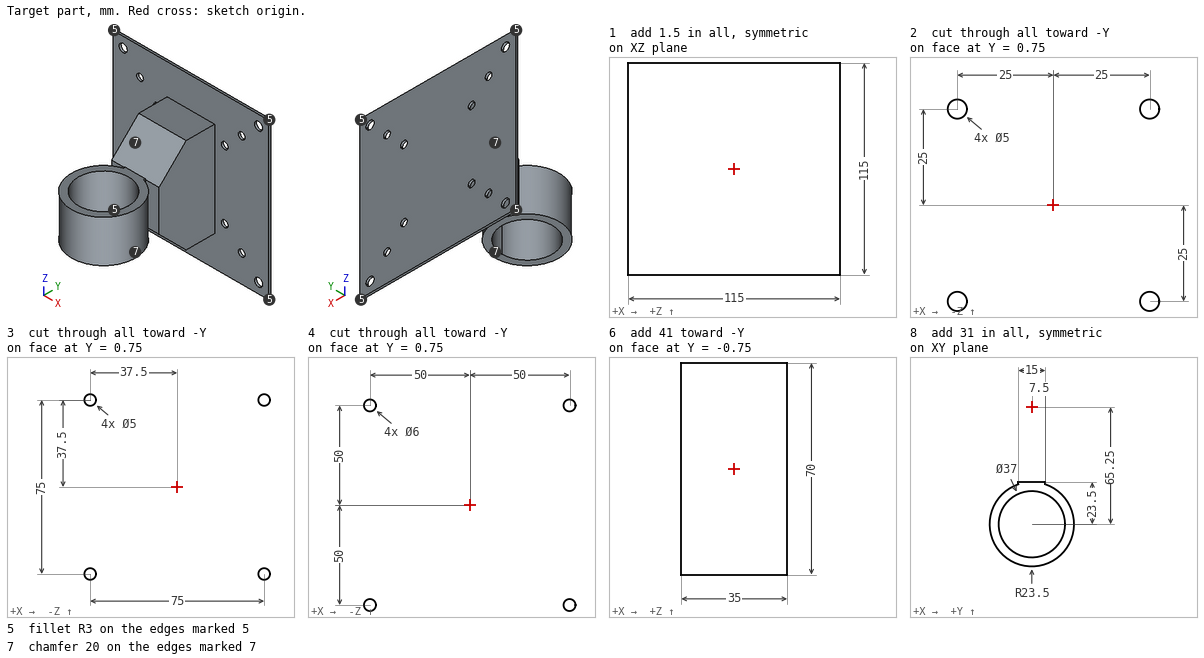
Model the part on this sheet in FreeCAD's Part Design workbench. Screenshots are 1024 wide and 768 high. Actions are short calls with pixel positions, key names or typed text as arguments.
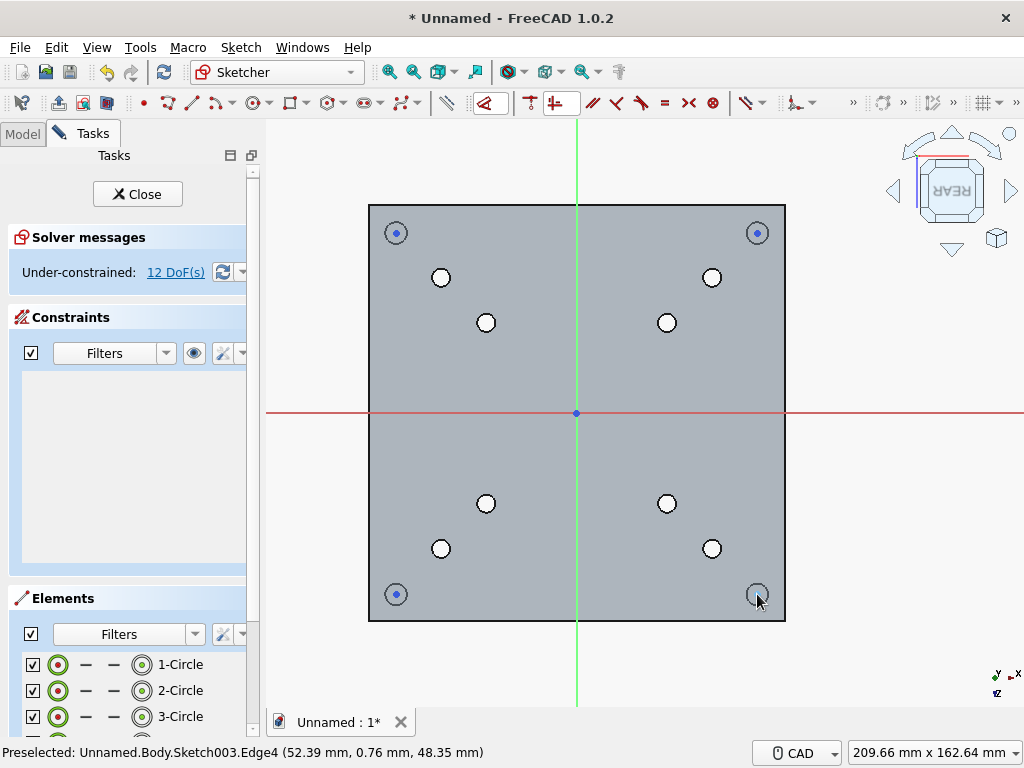
scroll(404, 225, up, 2)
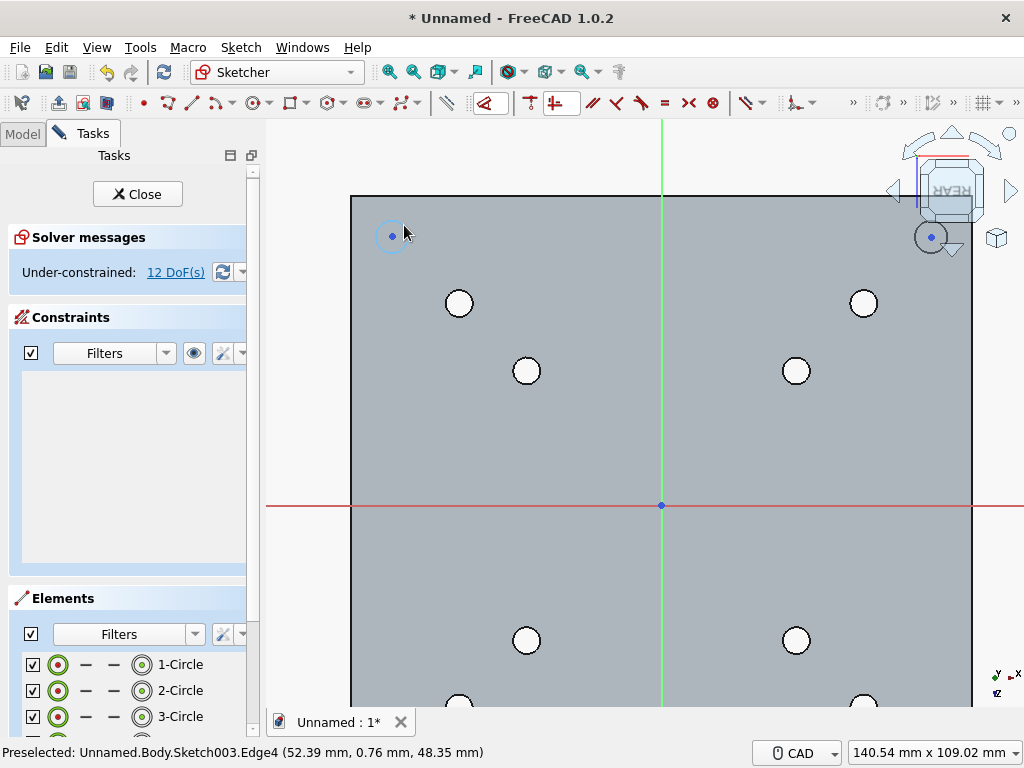
click(403, 225)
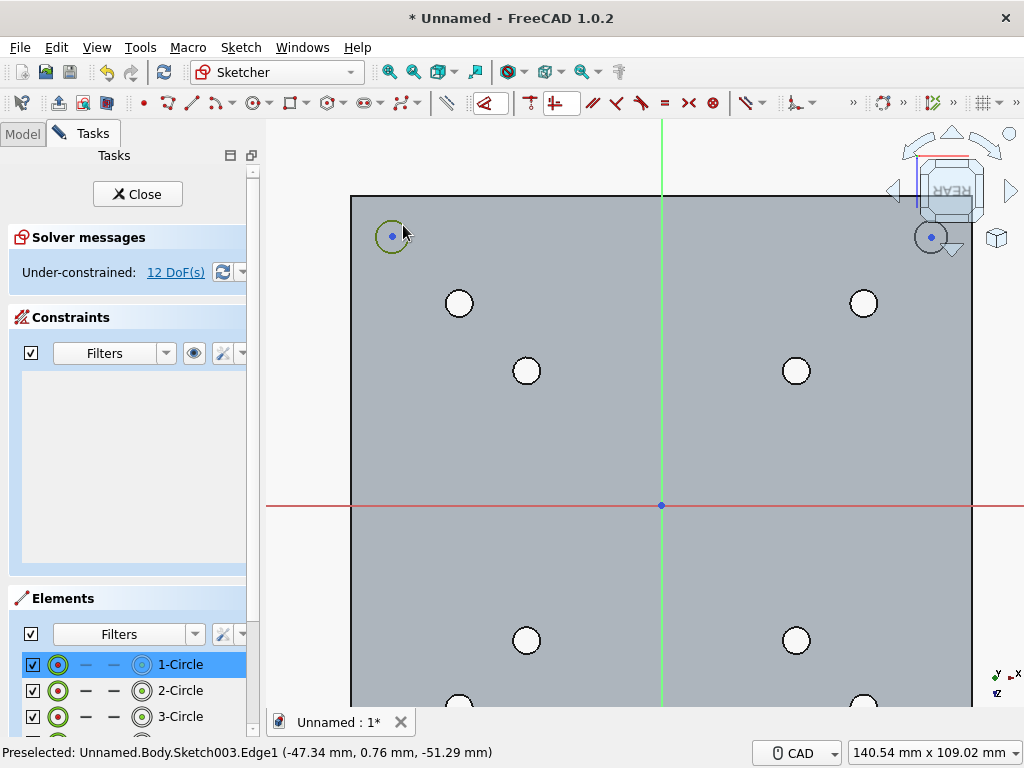
scroll(404, 224, down, 2)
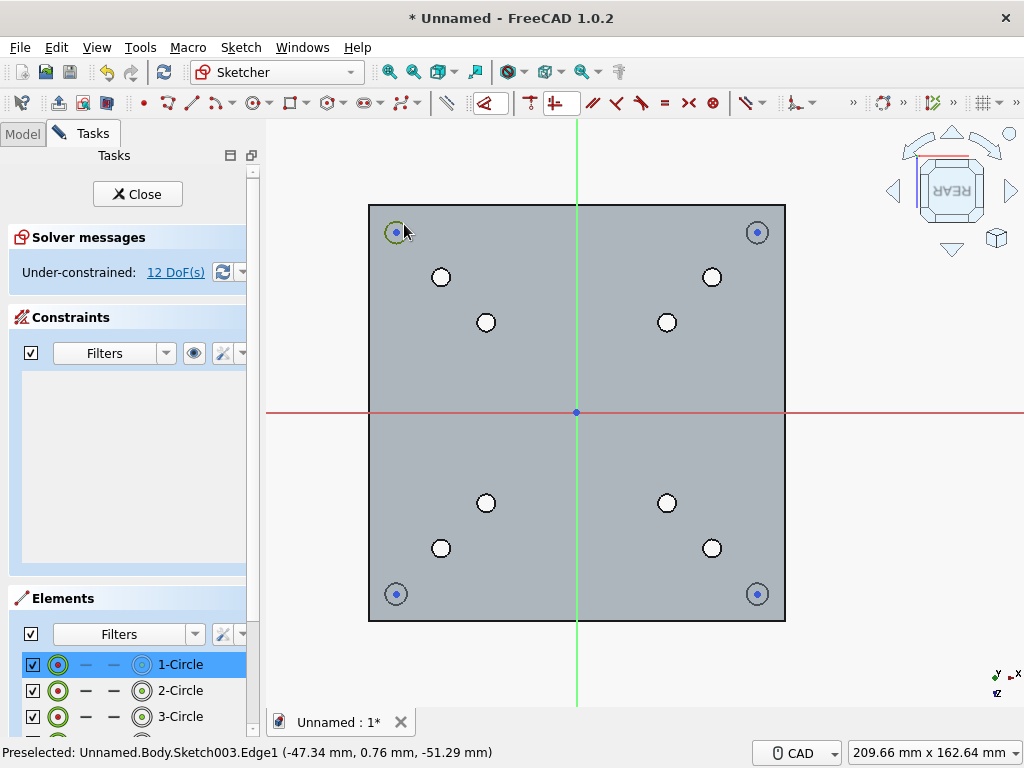
scroll(765, 225, up, 2)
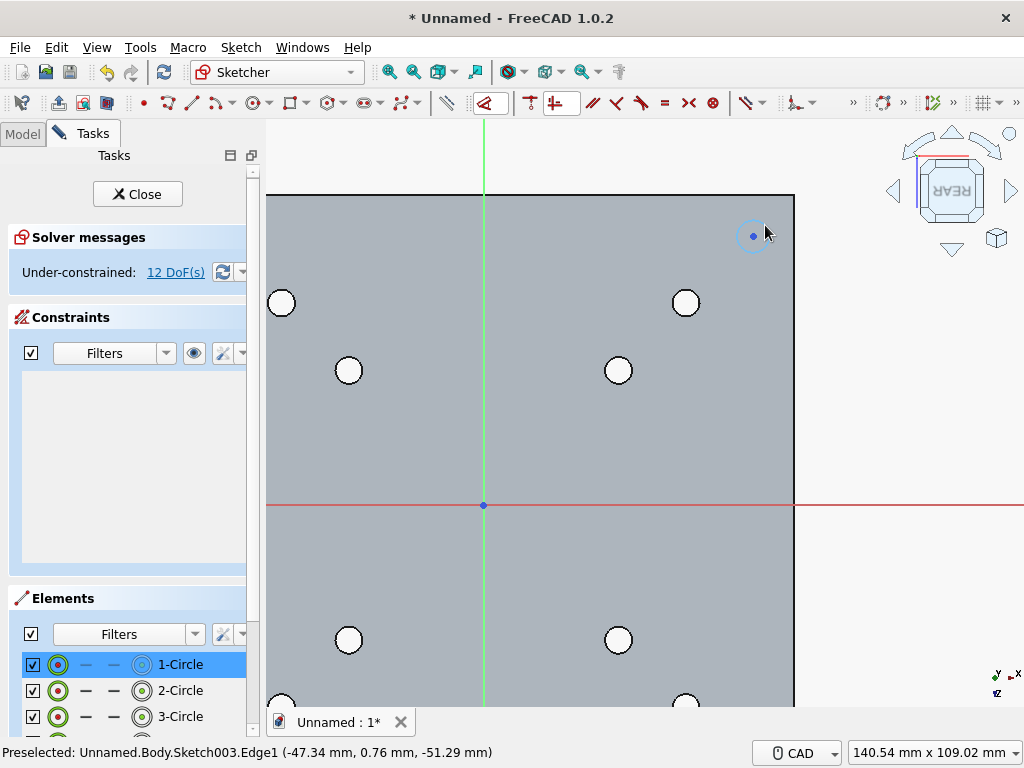
click(765, 225)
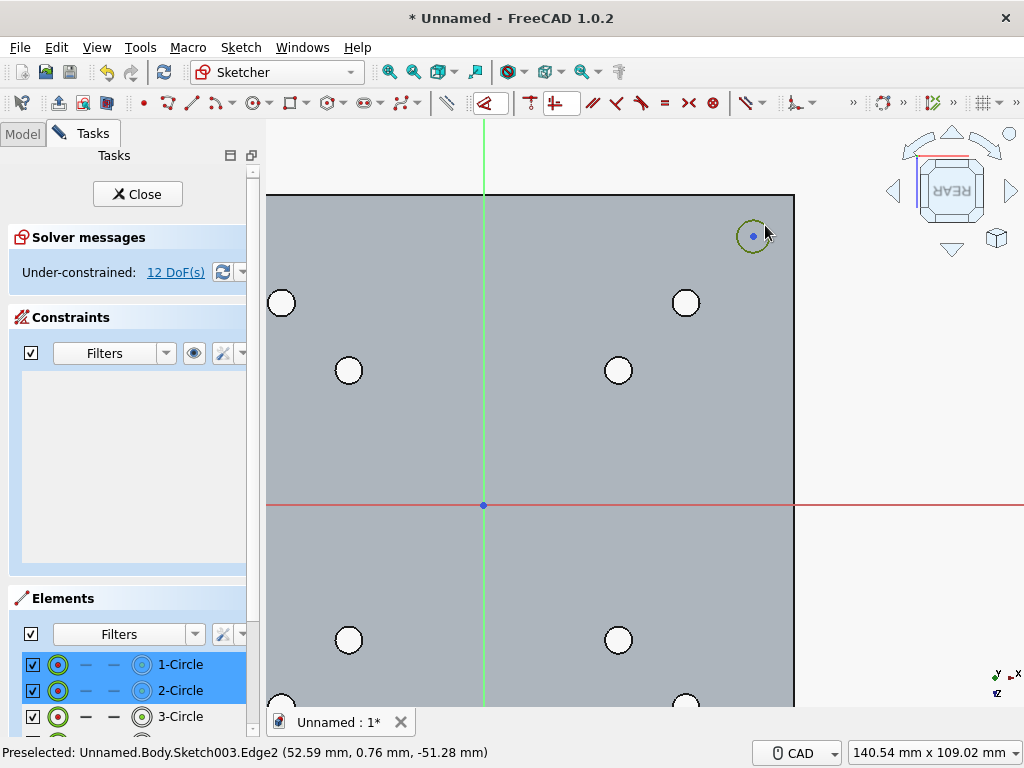
scroll(765, 225, down, 2)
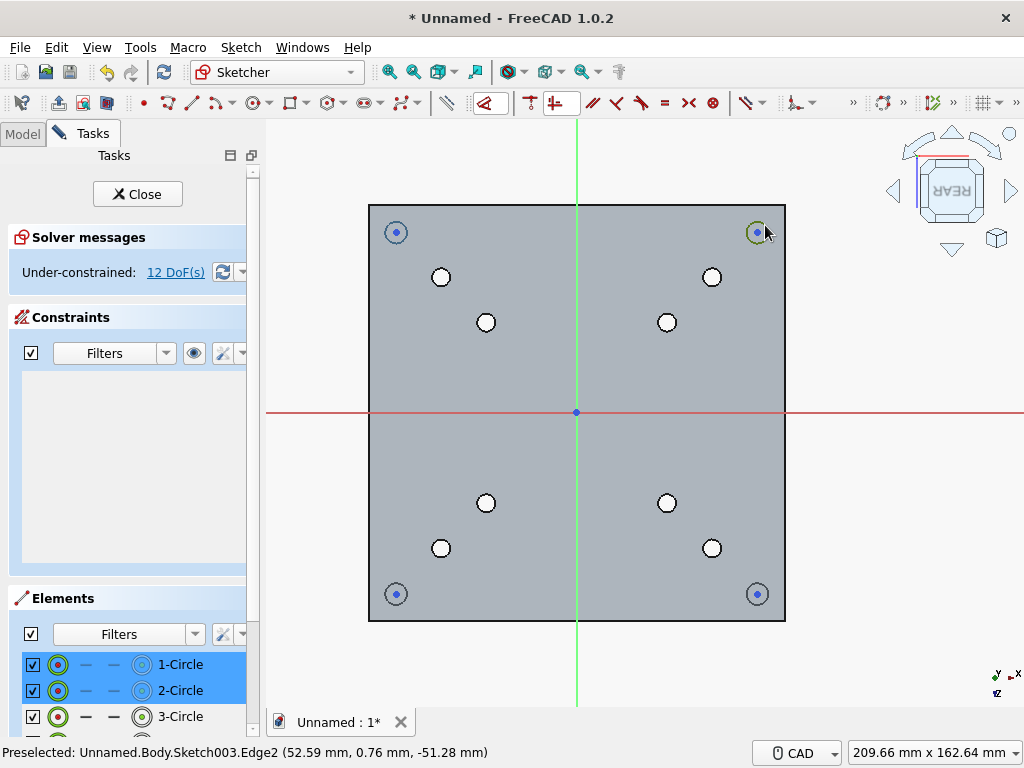
scroll(404, 586, up, 2)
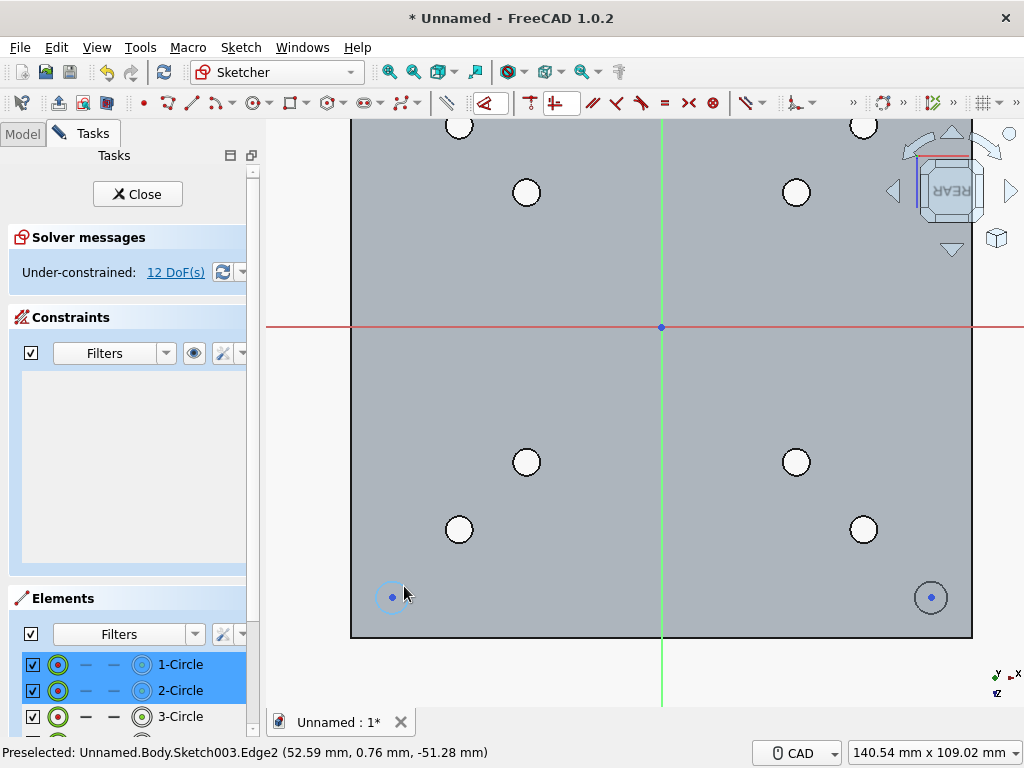
click(403, 586)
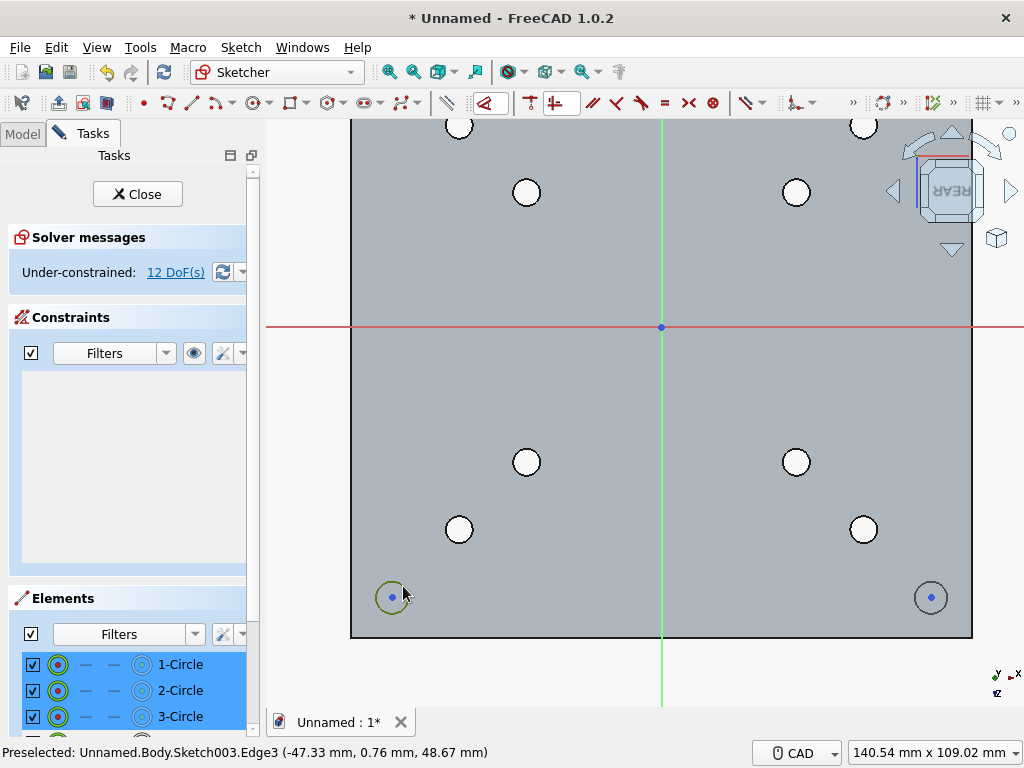
scroll(404, 587, down, 2)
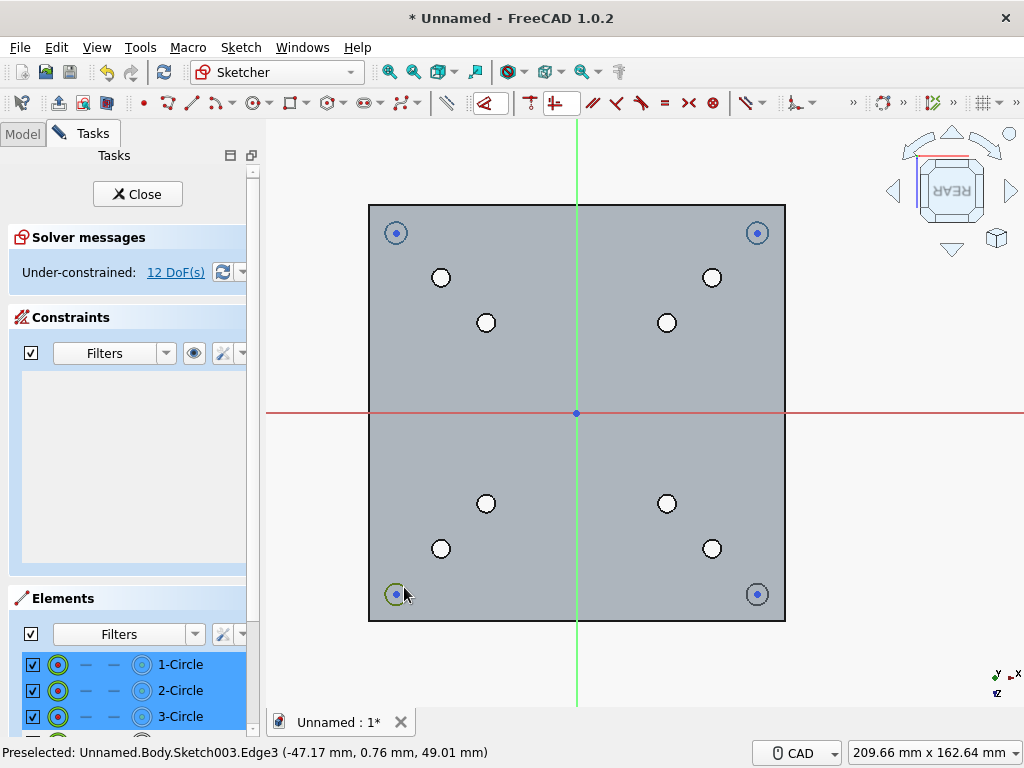
scroll(765, 587, up, 2)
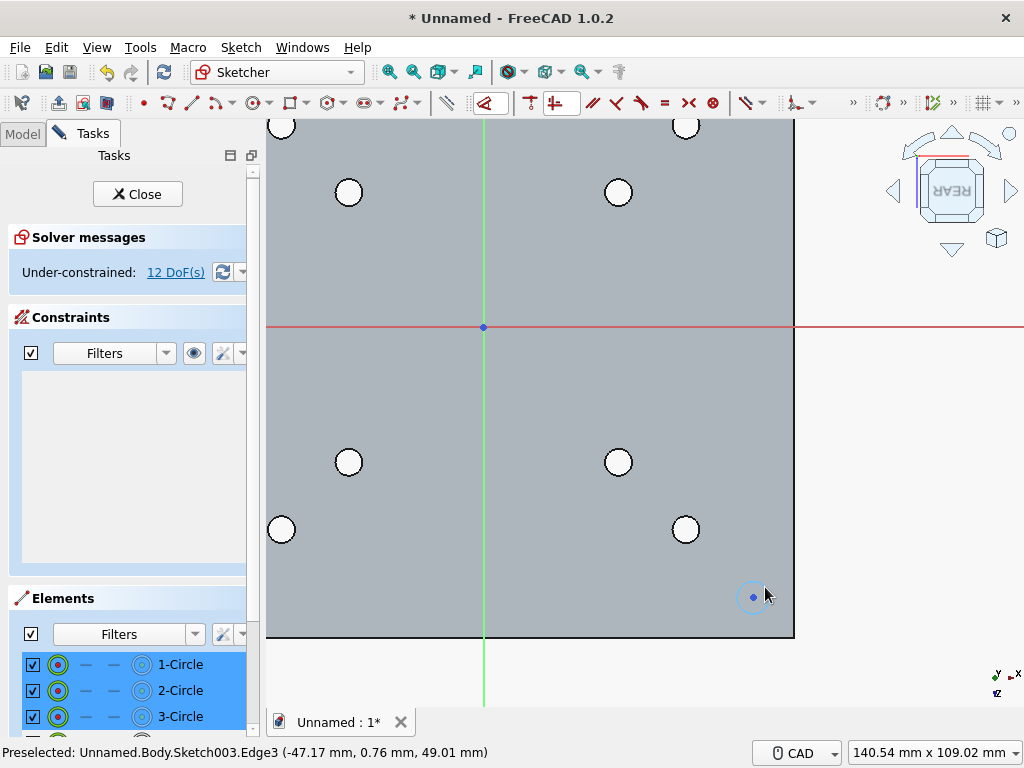
click(765, 586)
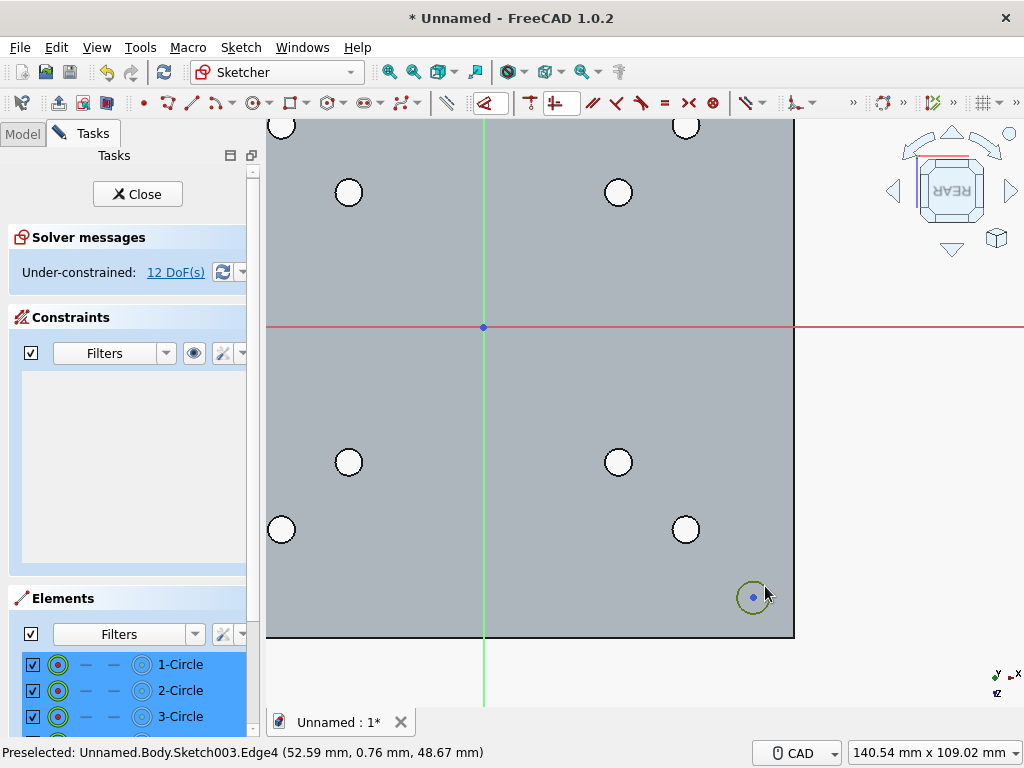
click(666, 104)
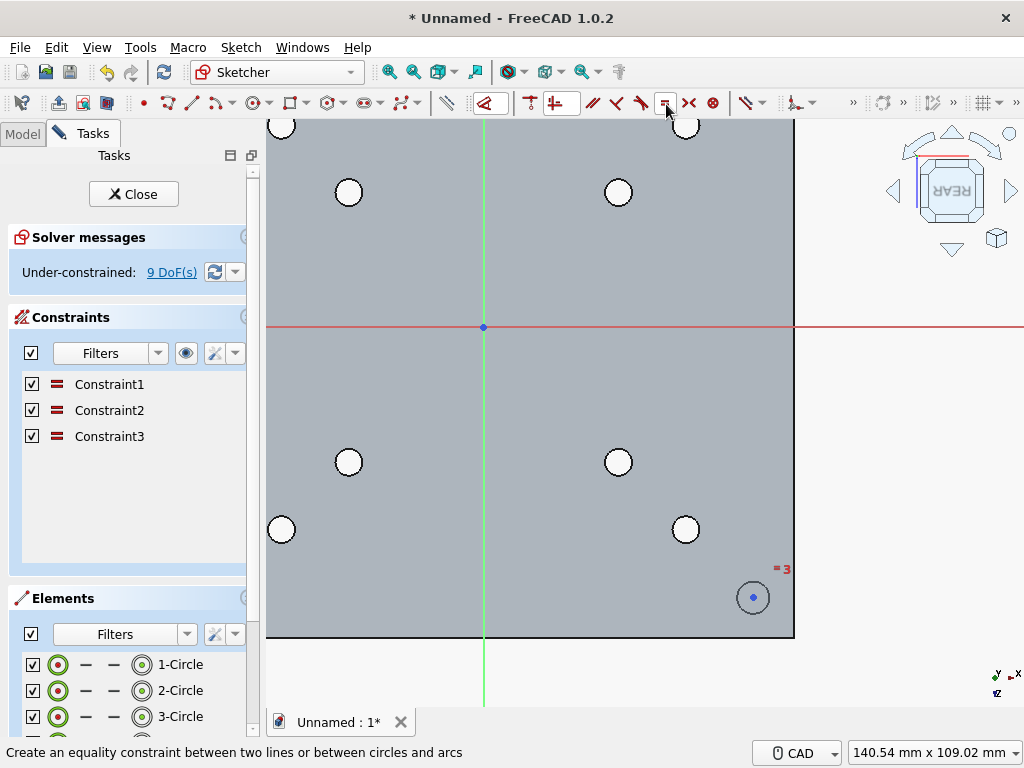
scroll(765, 587, down, 2)